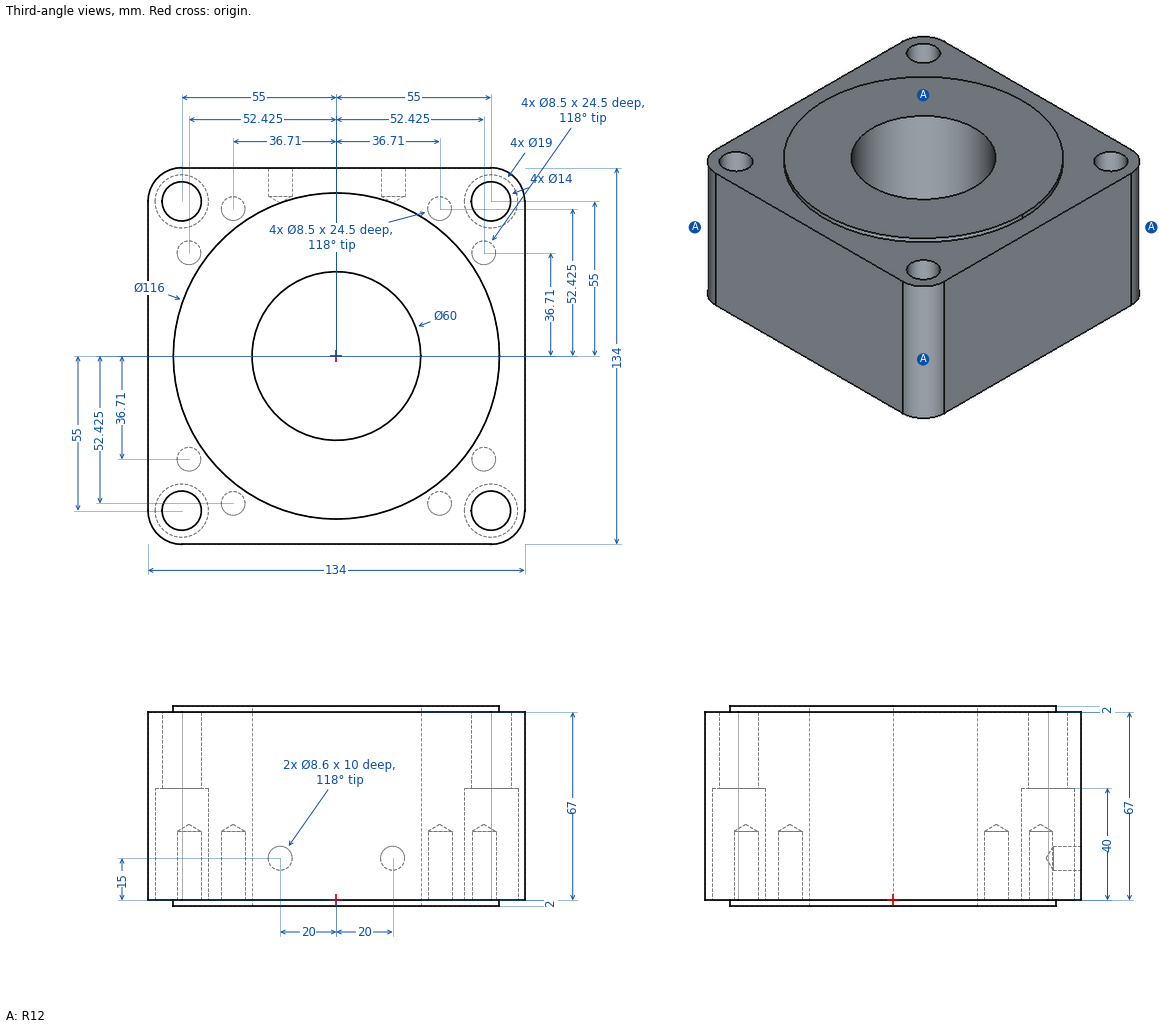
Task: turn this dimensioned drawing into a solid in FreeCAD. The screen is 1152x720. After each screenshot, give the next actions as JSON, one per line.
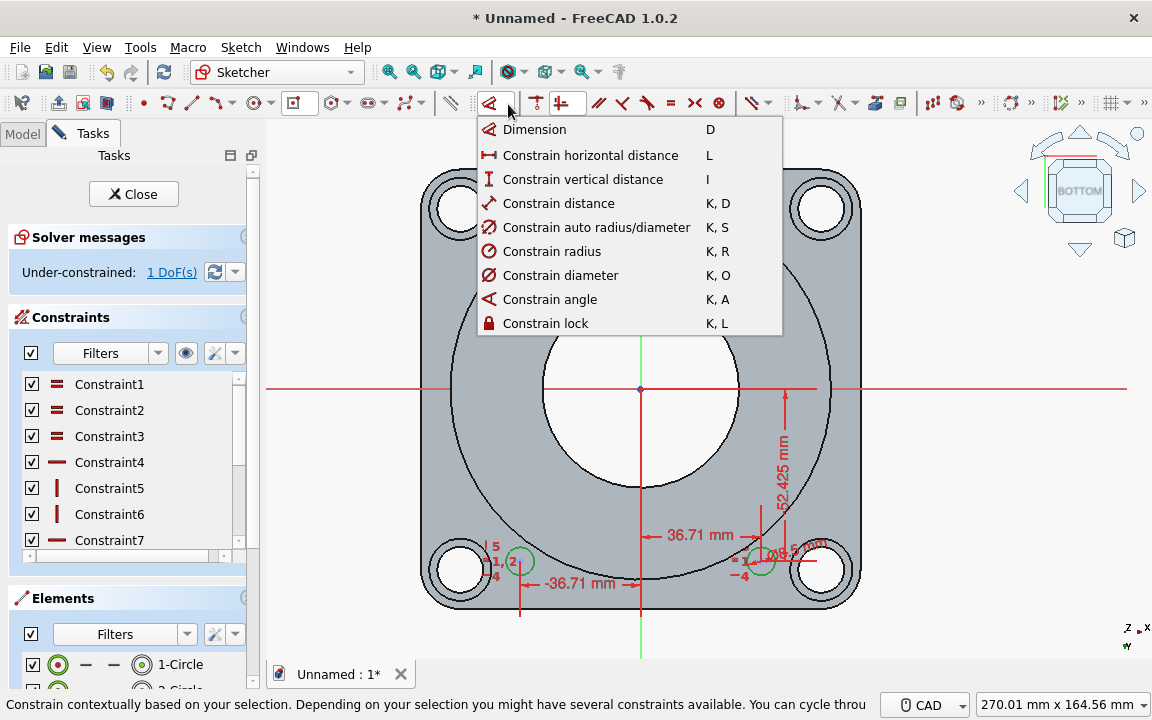
{"action": "left_click", "coordinate": [630, 179]}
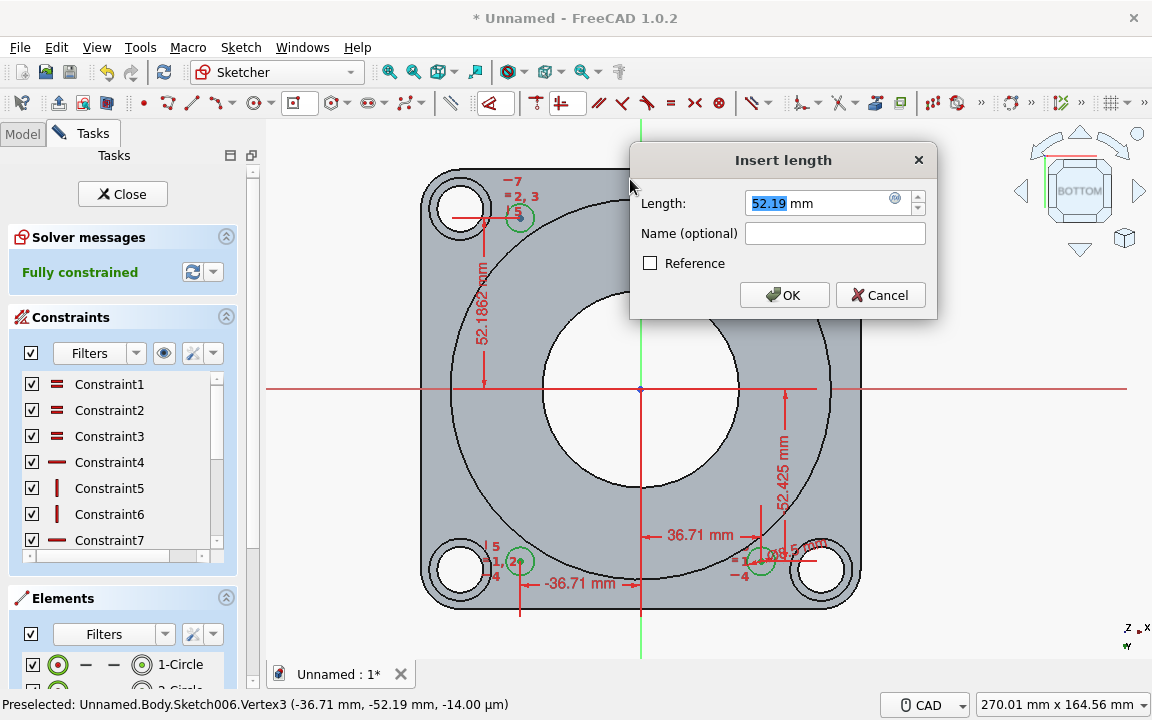
{"action": "type", "text": "52.425"}
{"action": "key", "text": "Return"}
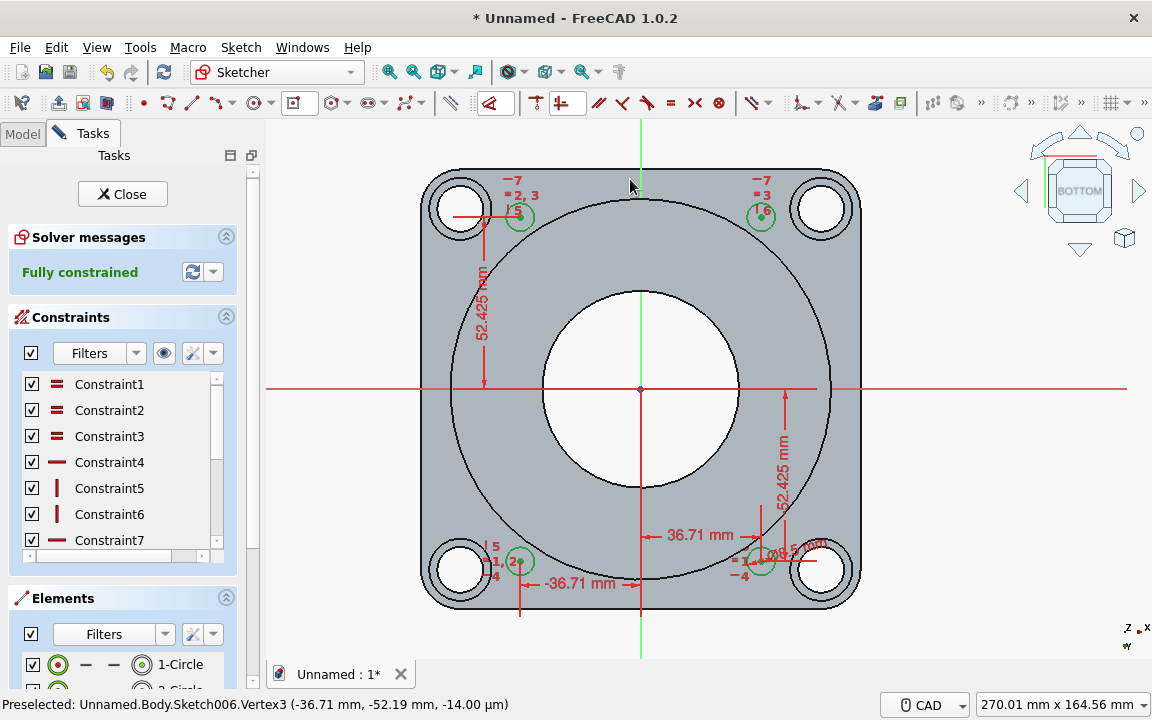
{"action": "left_click", "coordinate": [123, 194]}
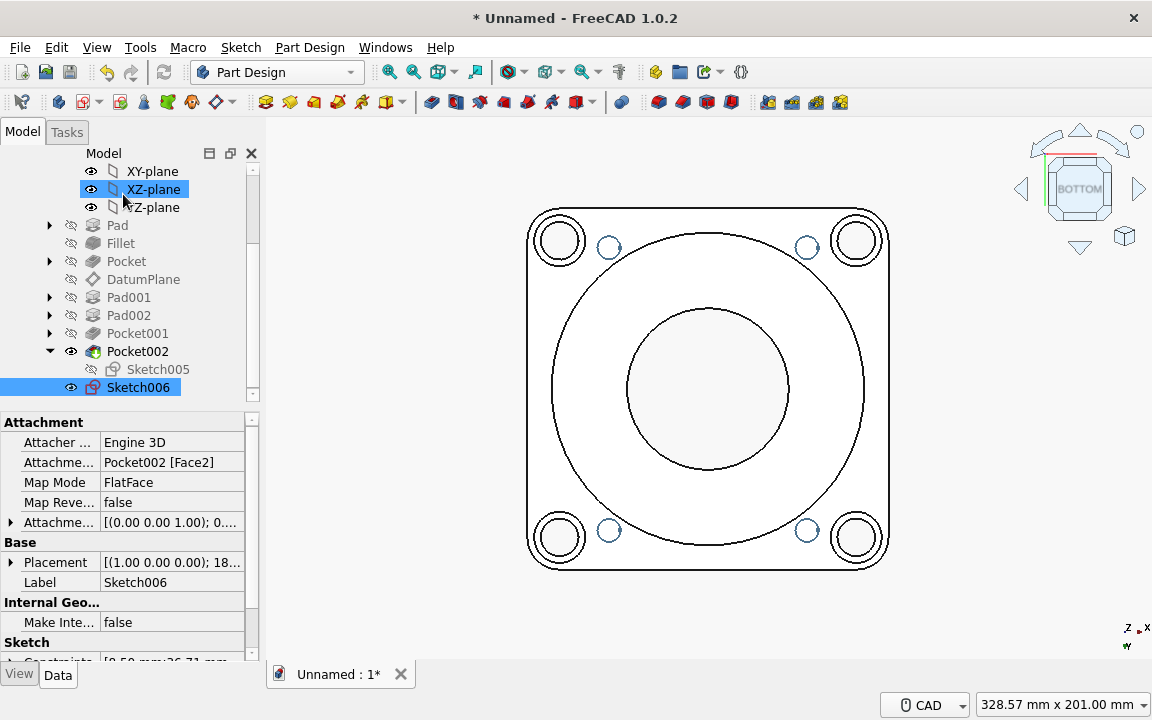
{"action": "left_click", "coordinate": [456, 102]}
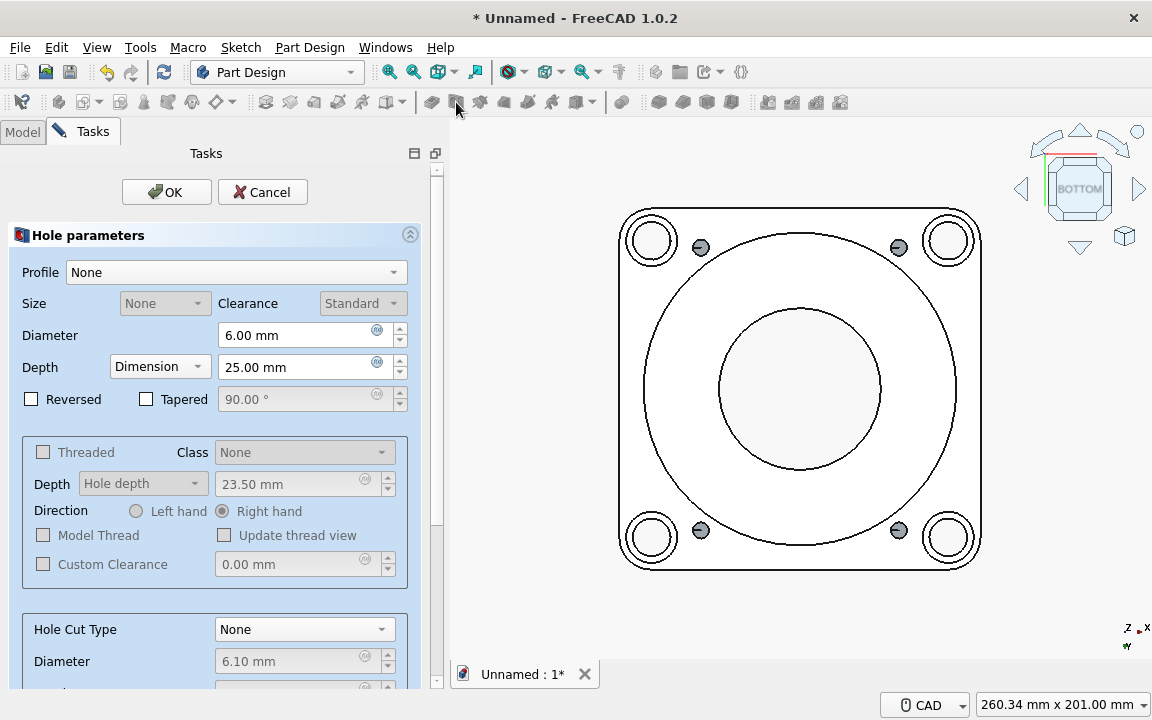
{"action": "triple_click", "coordinate": [305, 335]}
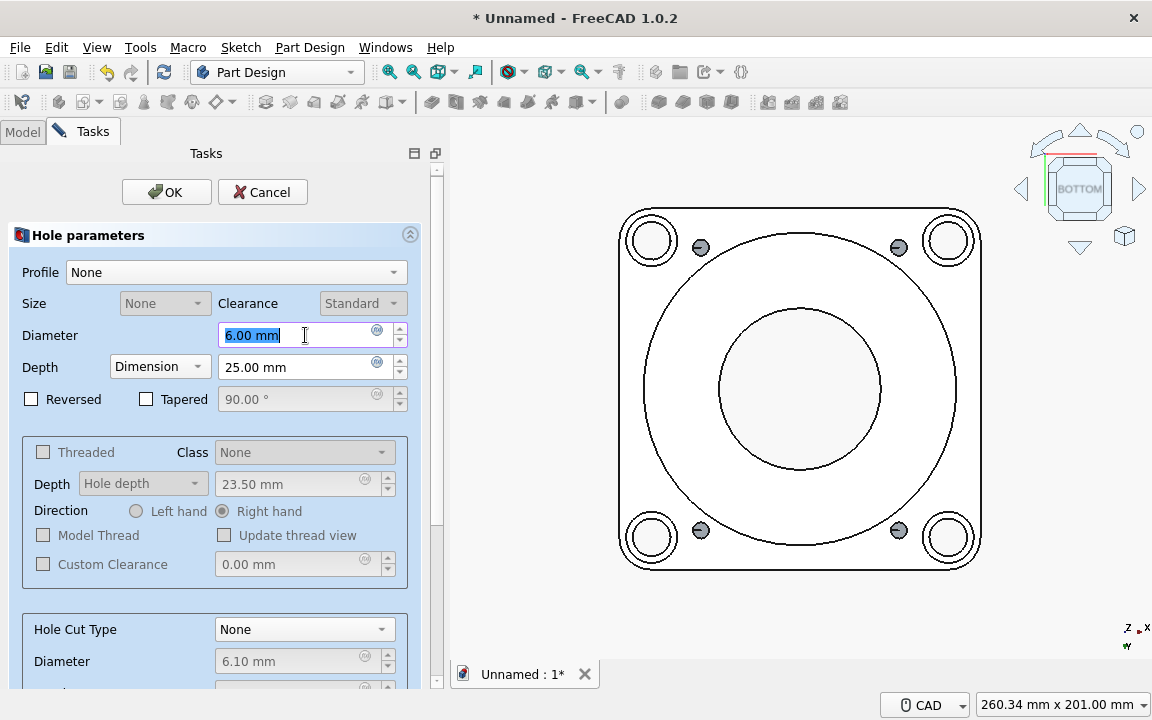
{"action": "type", "text": "8.5"}
{"action": "key", "text": "Tab"}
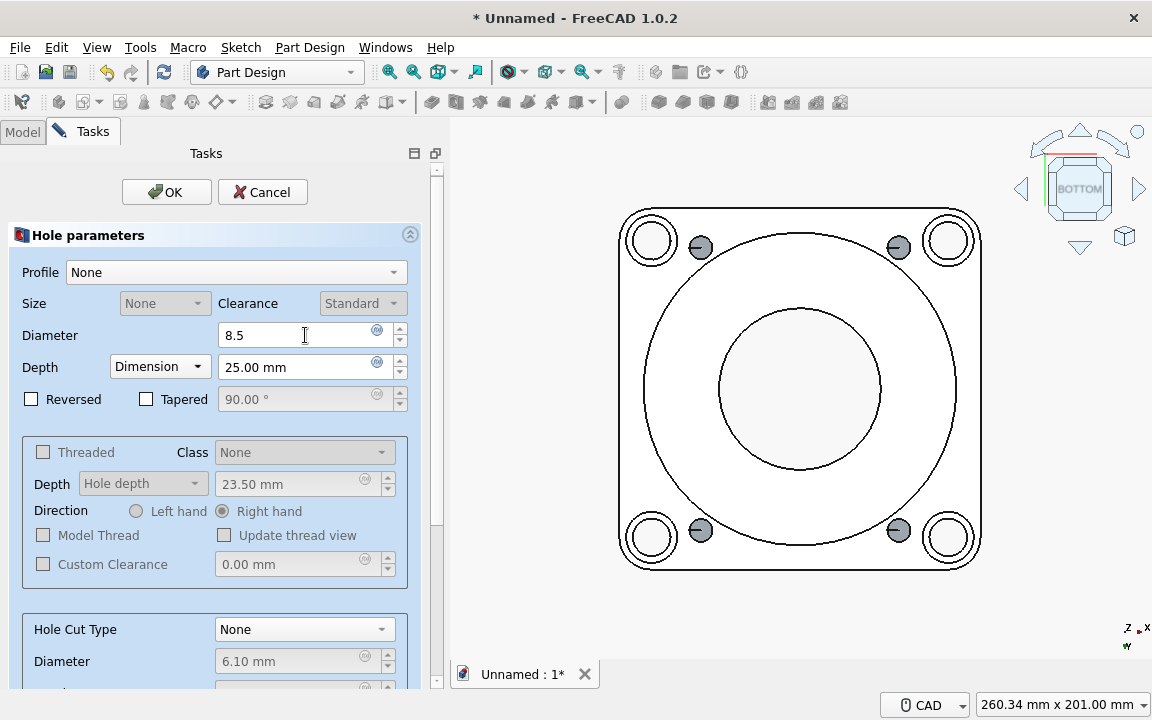
{"action": "triple_click", "coordinate": [305, 367]}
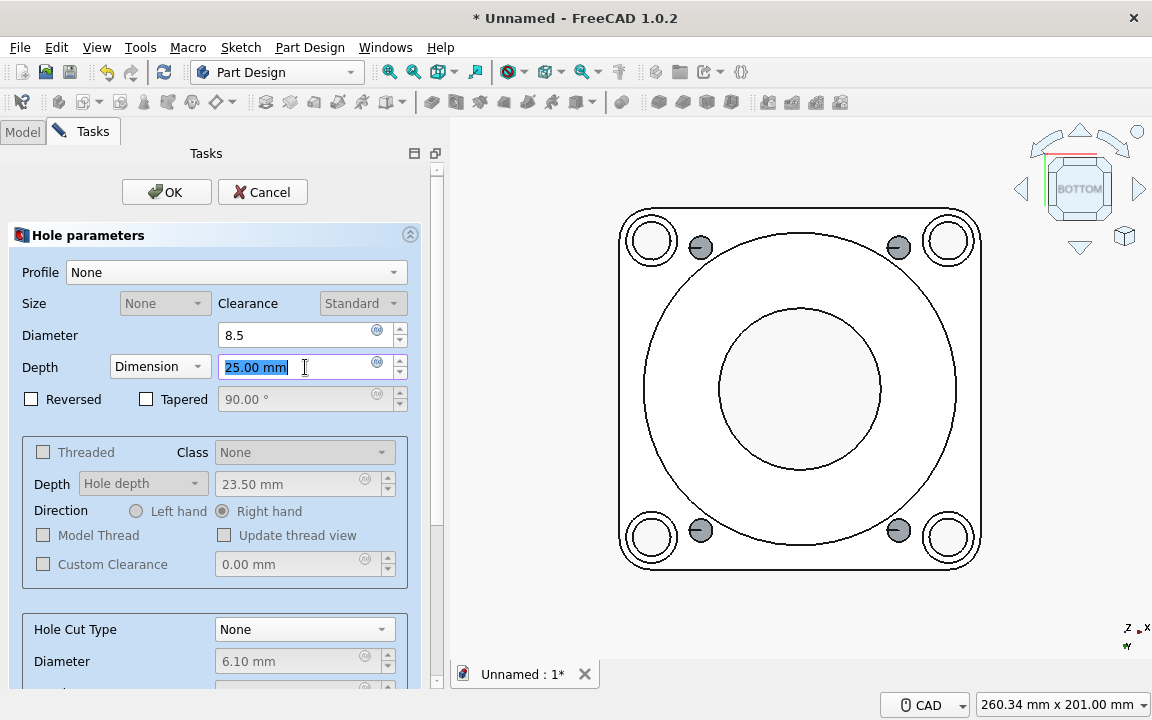
{"action": "type", "text": "24.5"}
{"action": "key", "text": "Tab"}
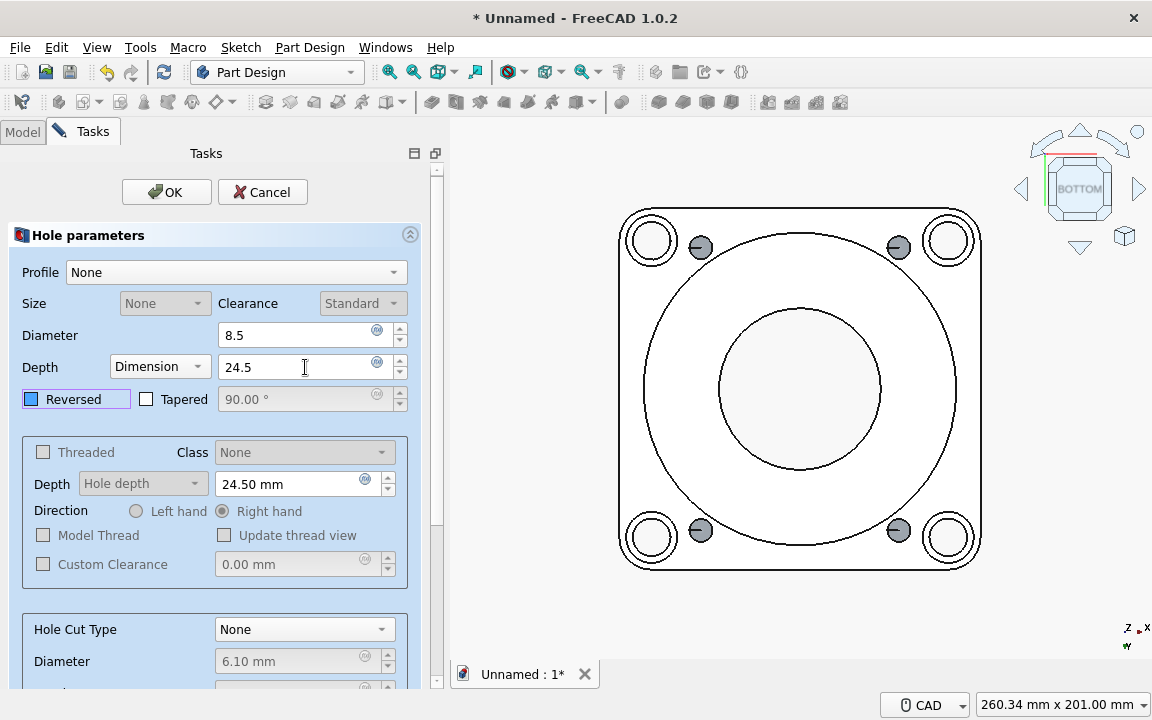
{"action": "left_click", "coordinate": [167, 192]}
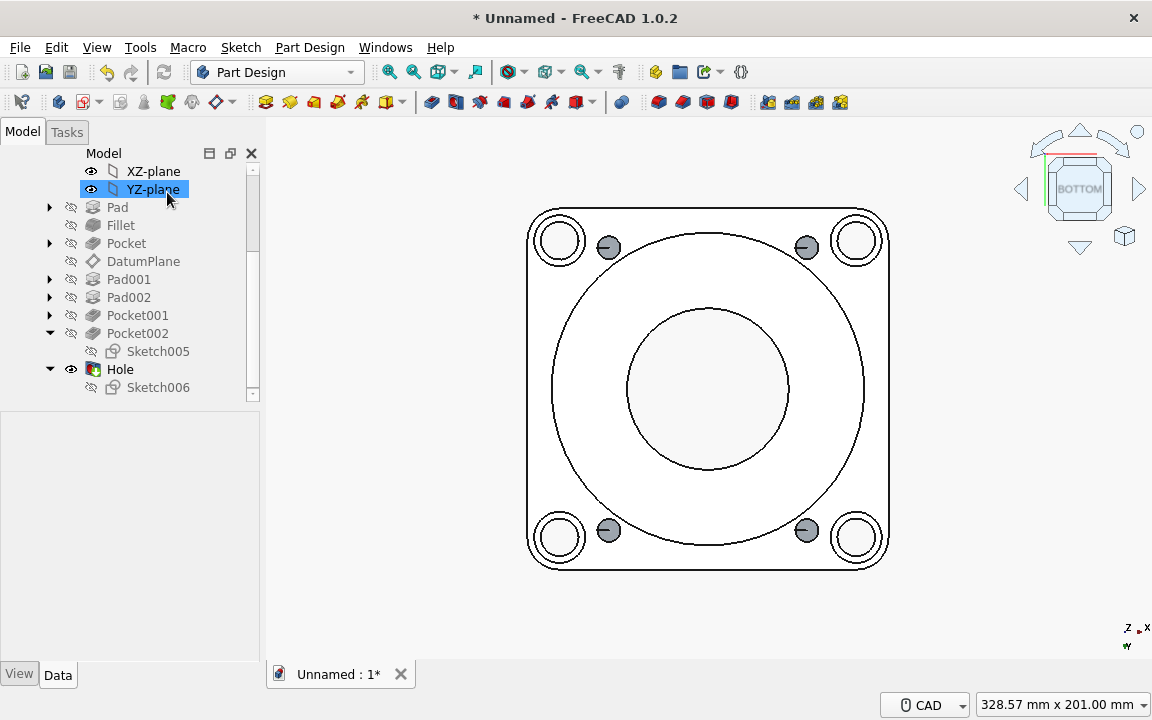
{"action": "left_click", "coordinate": [863, 285]}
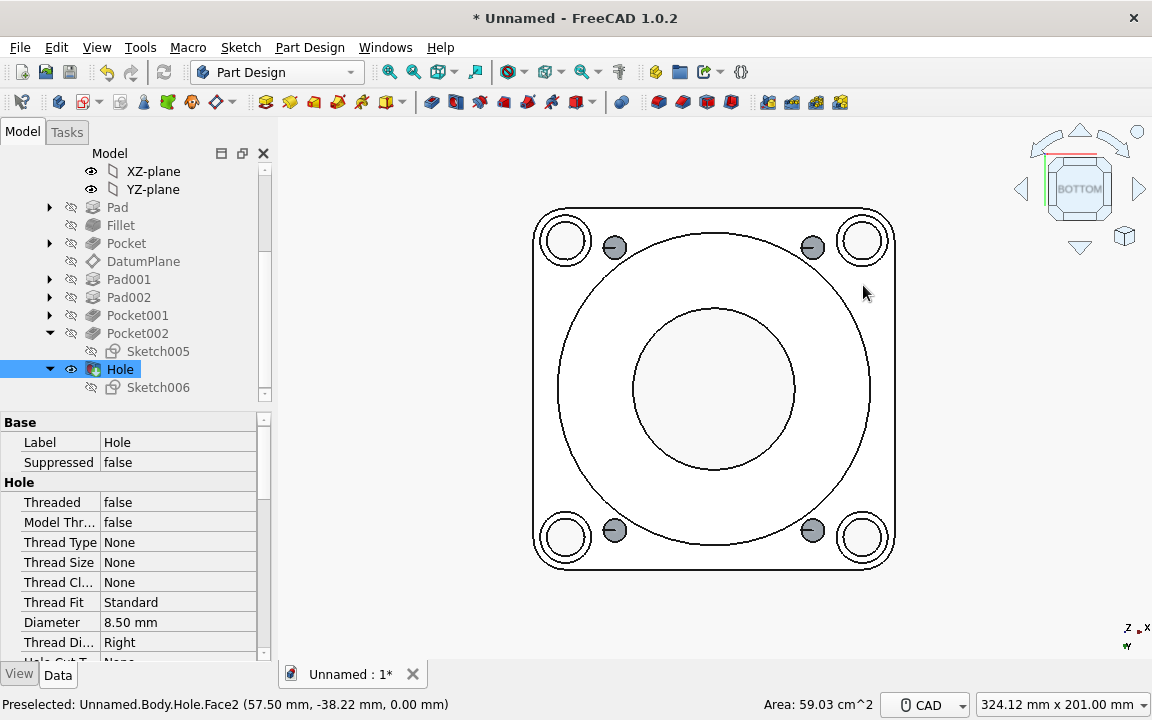
{"action": "left_click", "coordinate": [84, 102]}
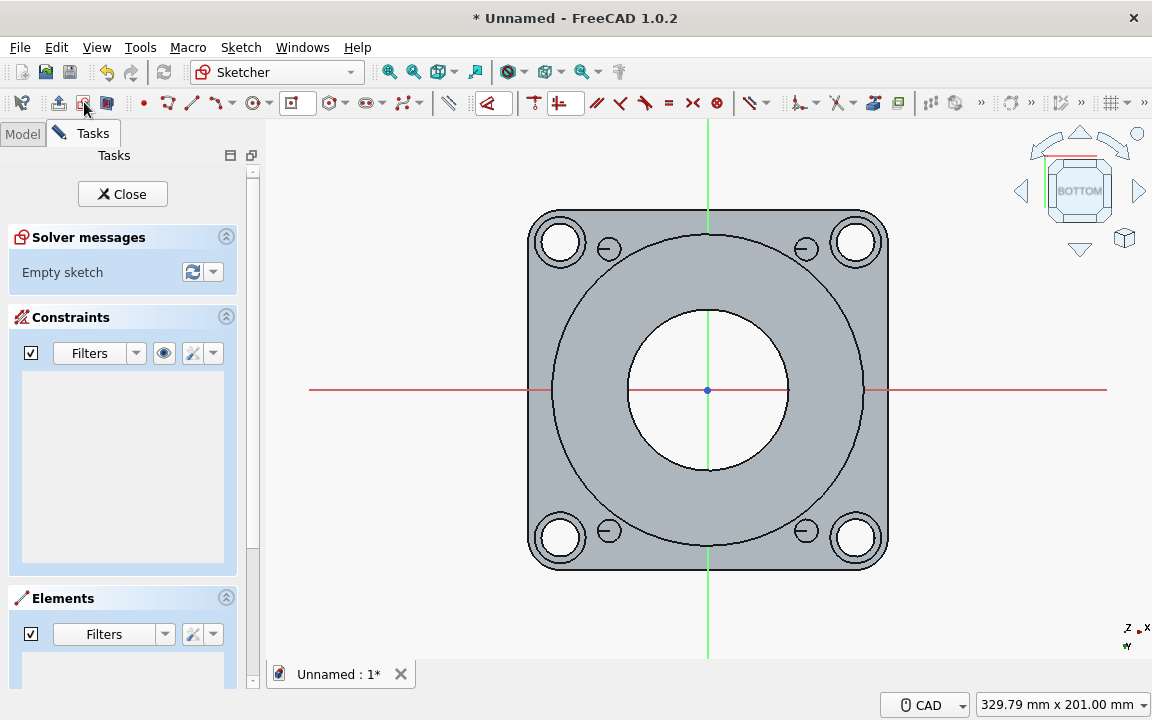
{"action": "left_click", "coordinate": [108, 104]}